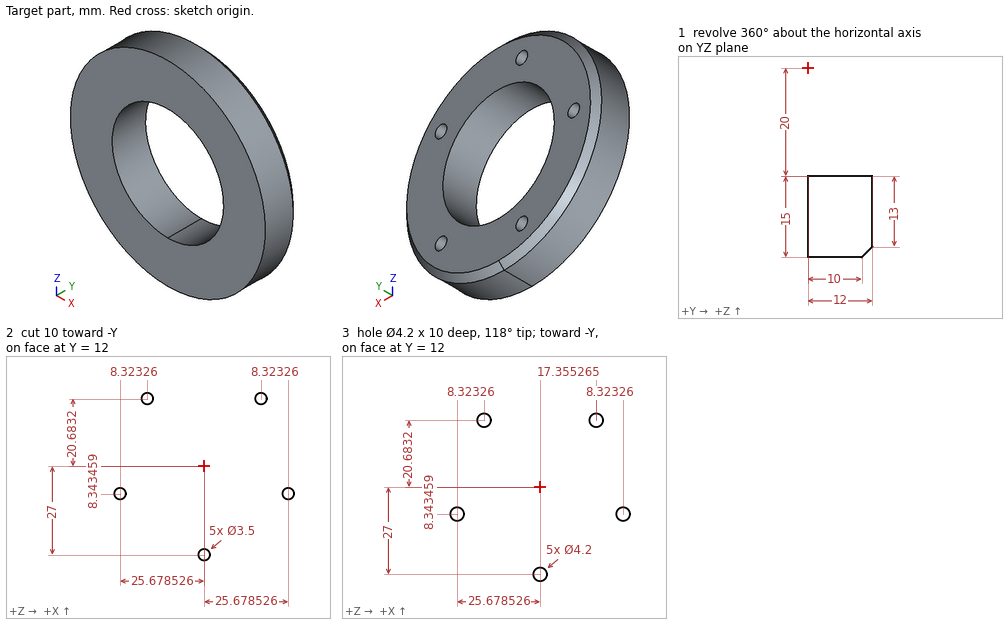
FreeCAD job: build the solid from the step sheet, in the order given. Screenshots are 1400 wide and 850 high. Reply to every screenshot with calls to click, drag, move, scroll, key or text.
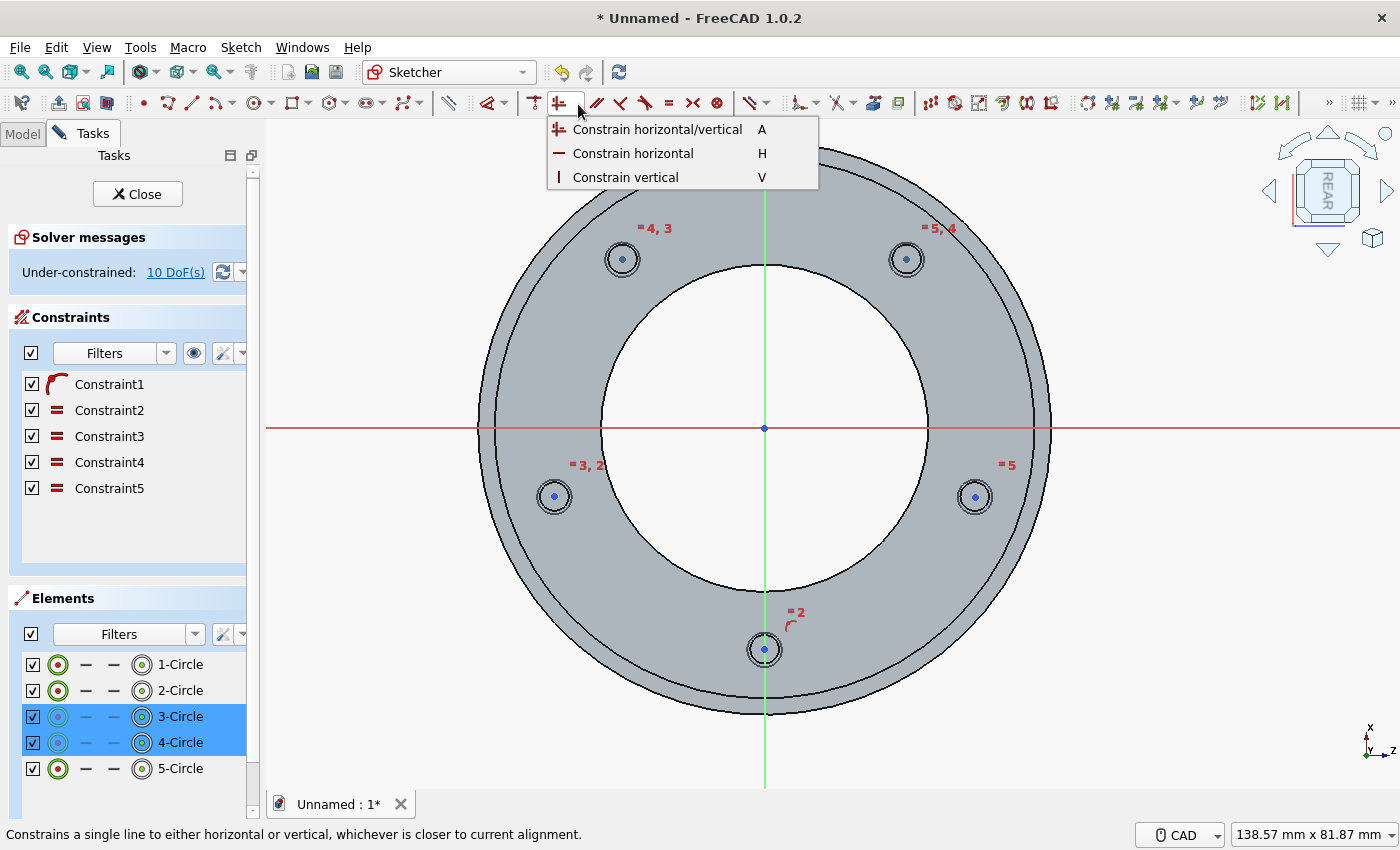
click(683, 153)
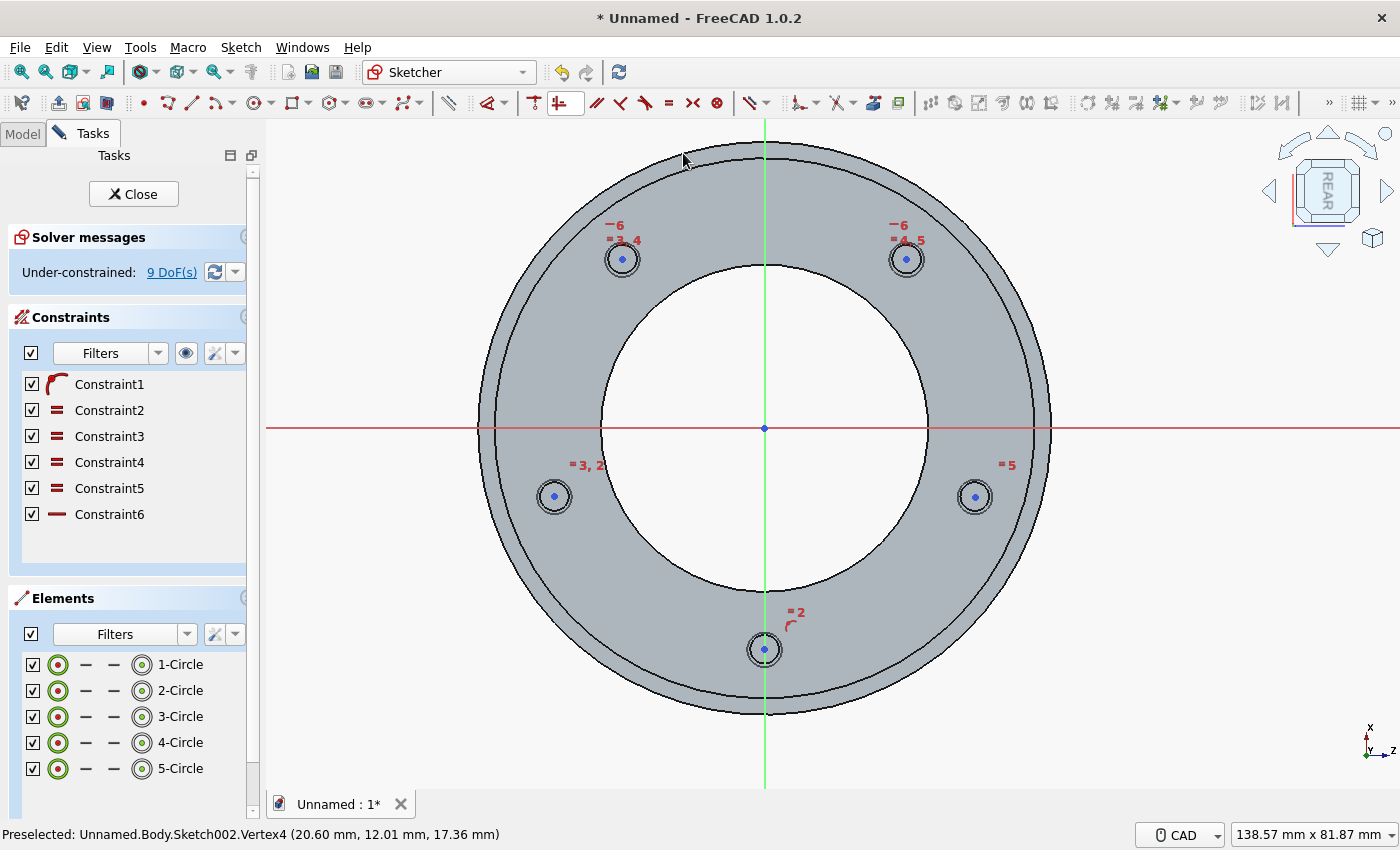
click(554, 497)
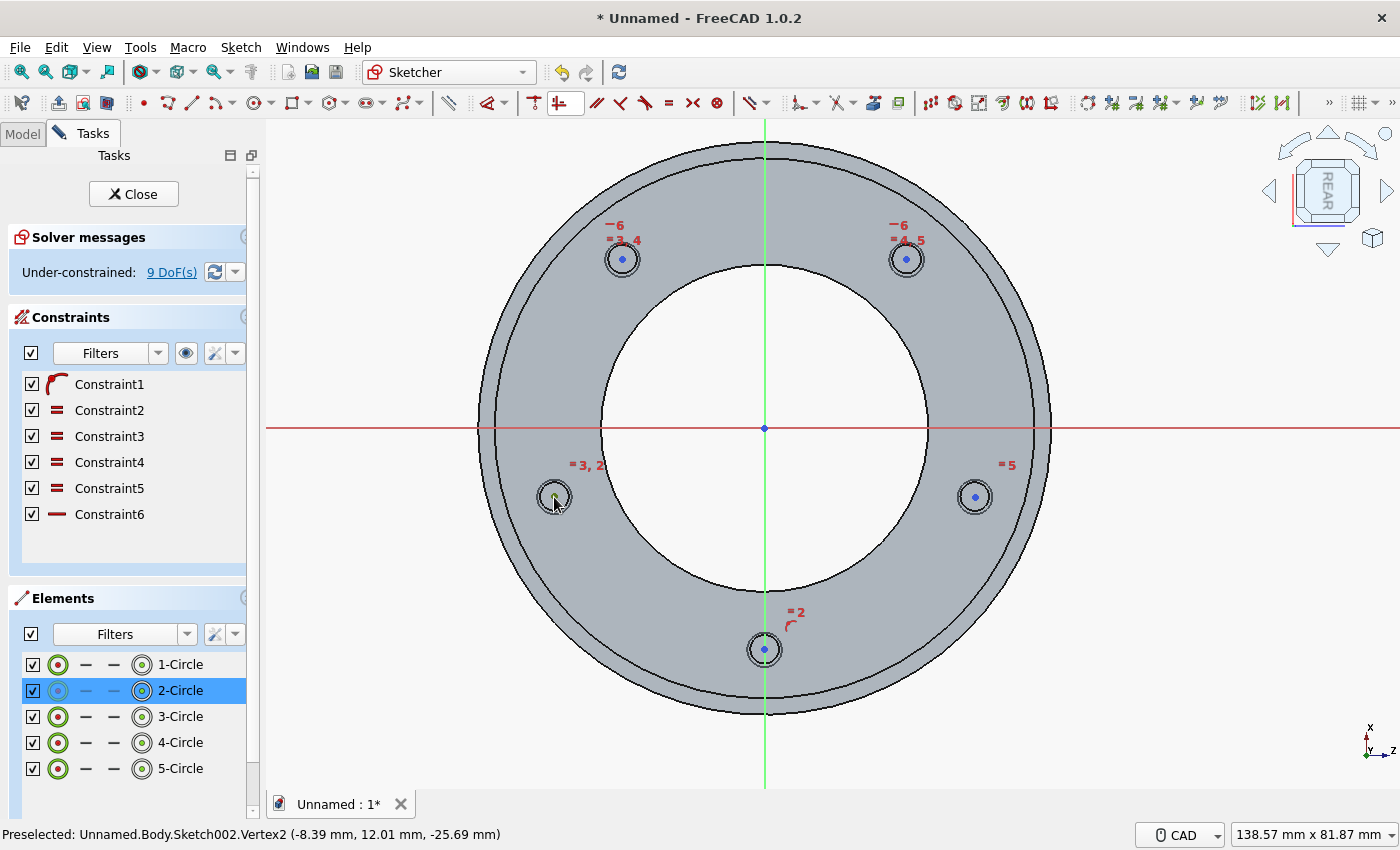
click(975, 497)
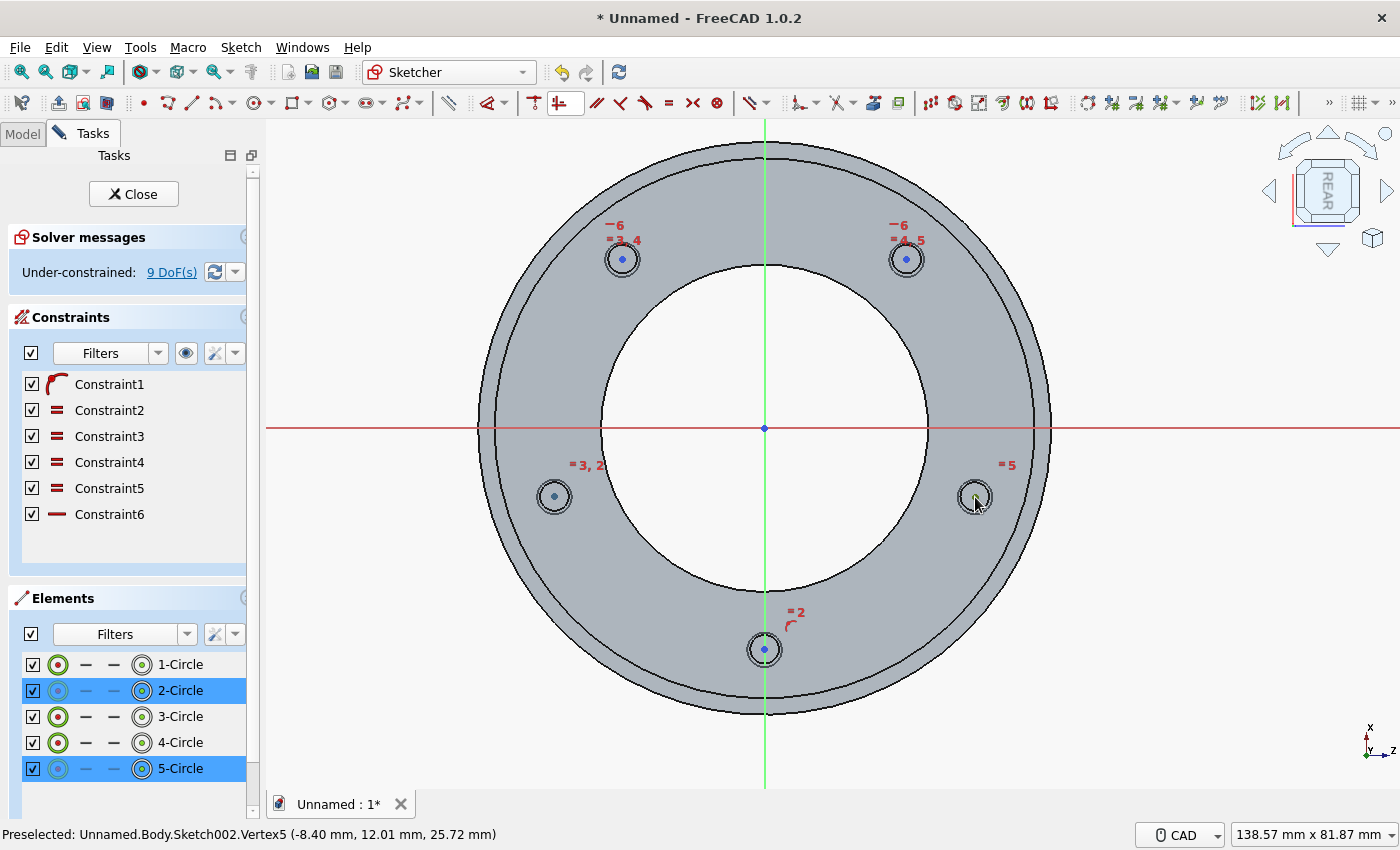
key(h)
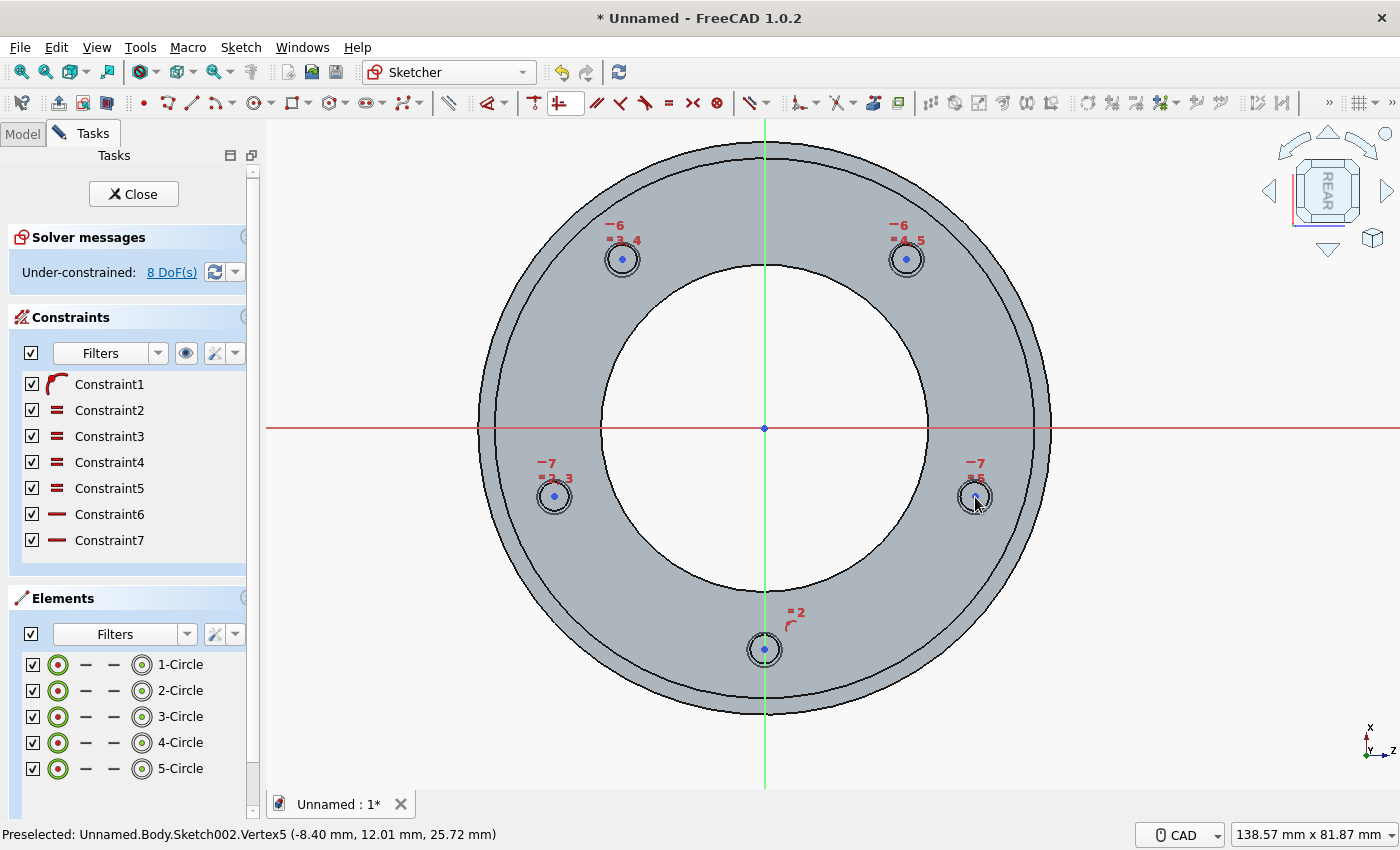
click(488, 104)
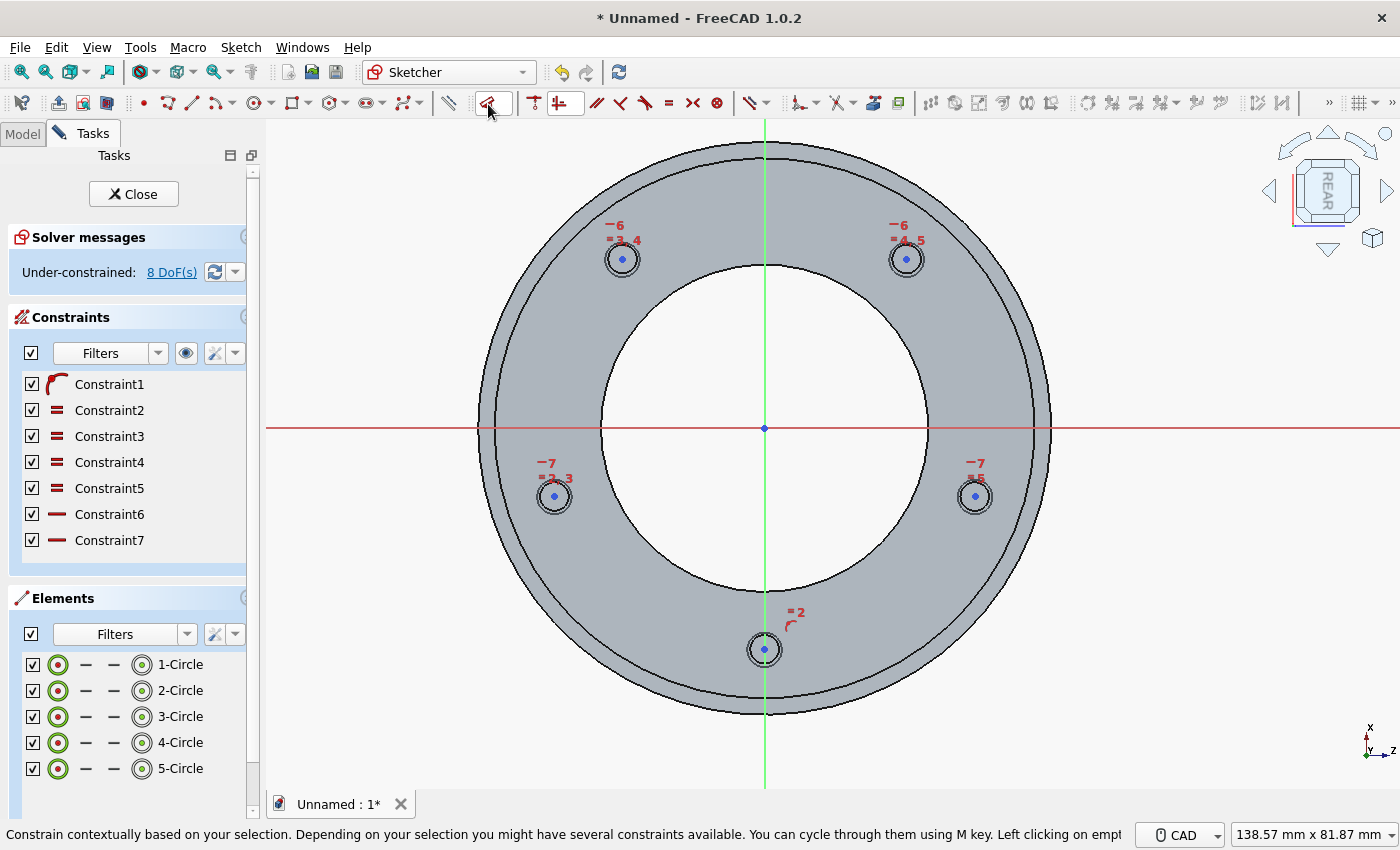
click(777, 638)
click(800, 616)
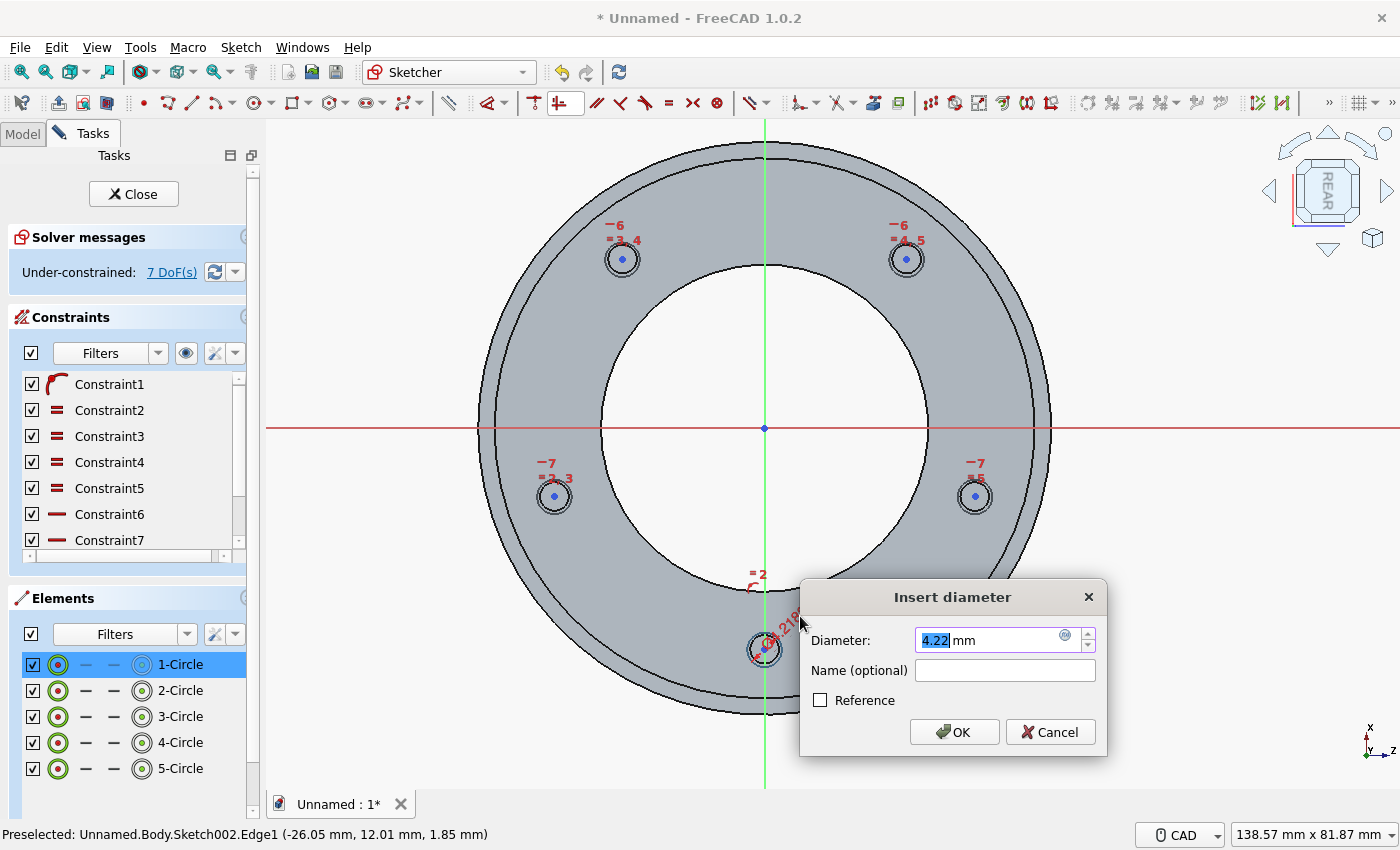
text(4.2)
key(Return)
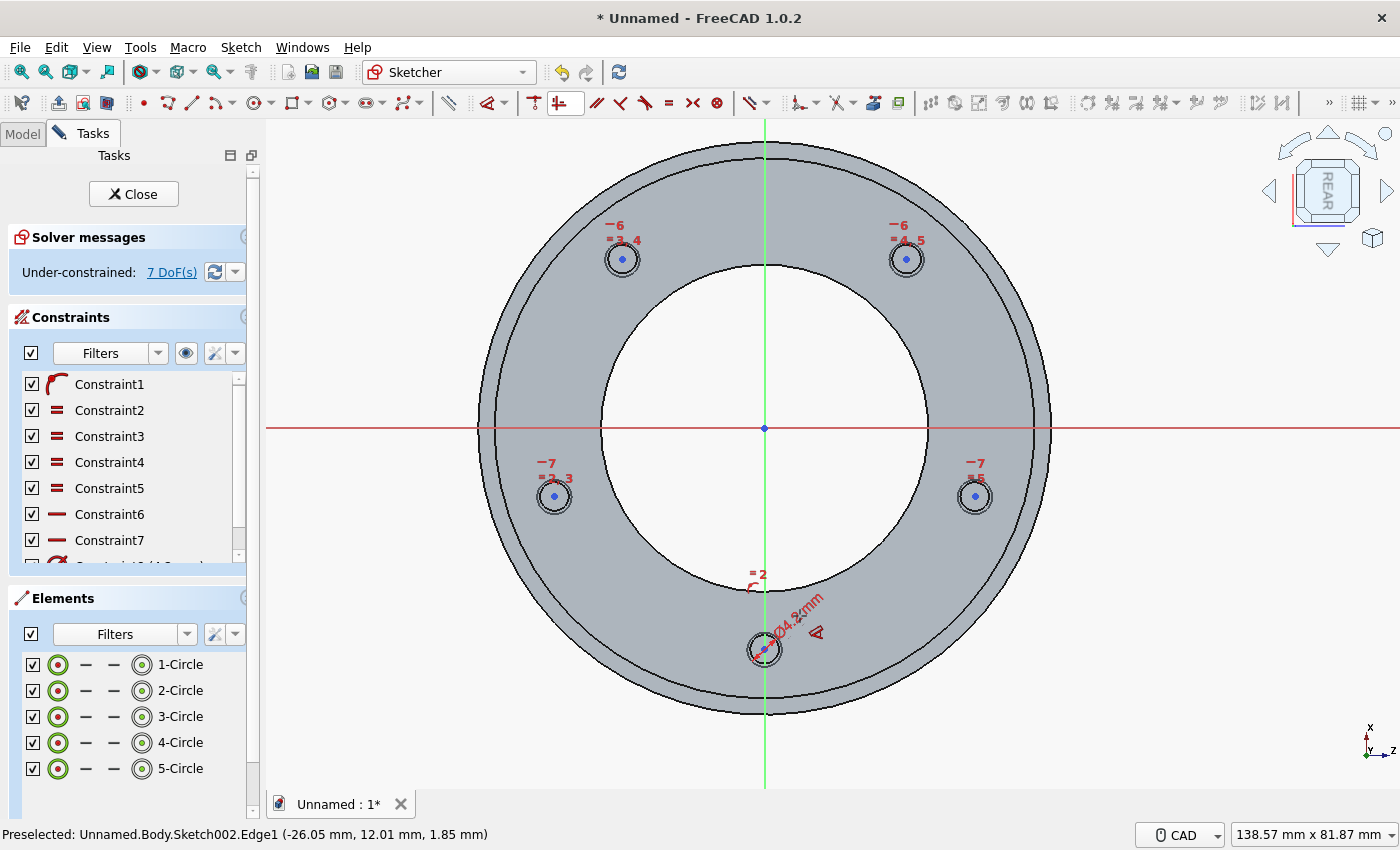
click(765, 650)
click(799, 539)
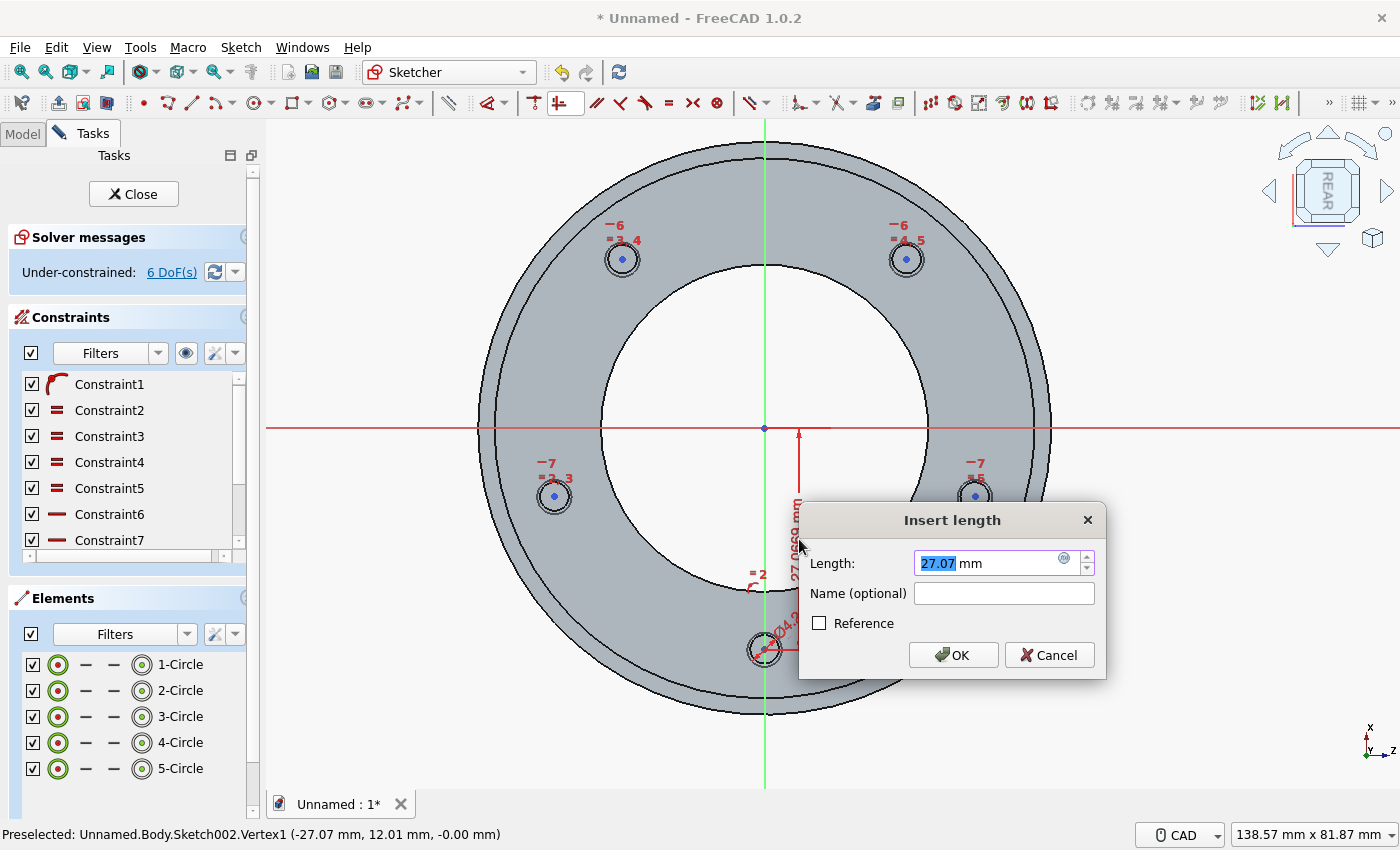
text(27)
key(Return)